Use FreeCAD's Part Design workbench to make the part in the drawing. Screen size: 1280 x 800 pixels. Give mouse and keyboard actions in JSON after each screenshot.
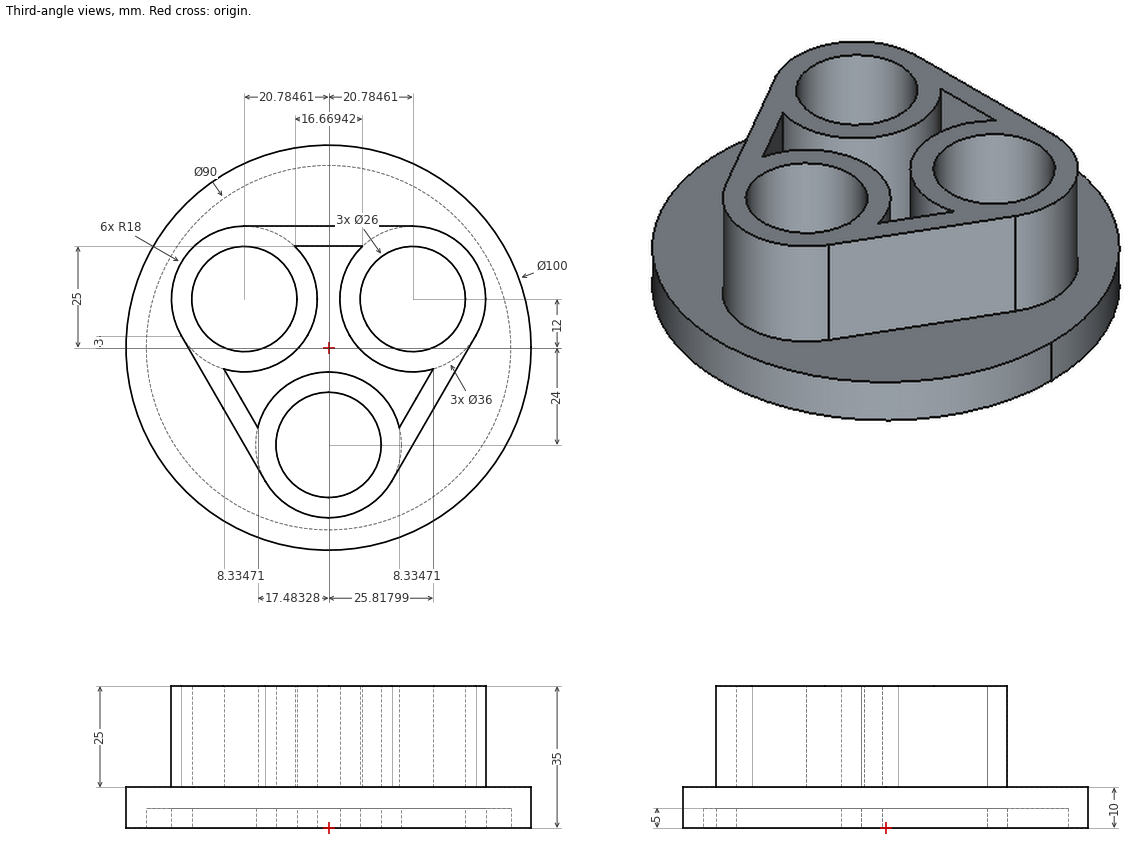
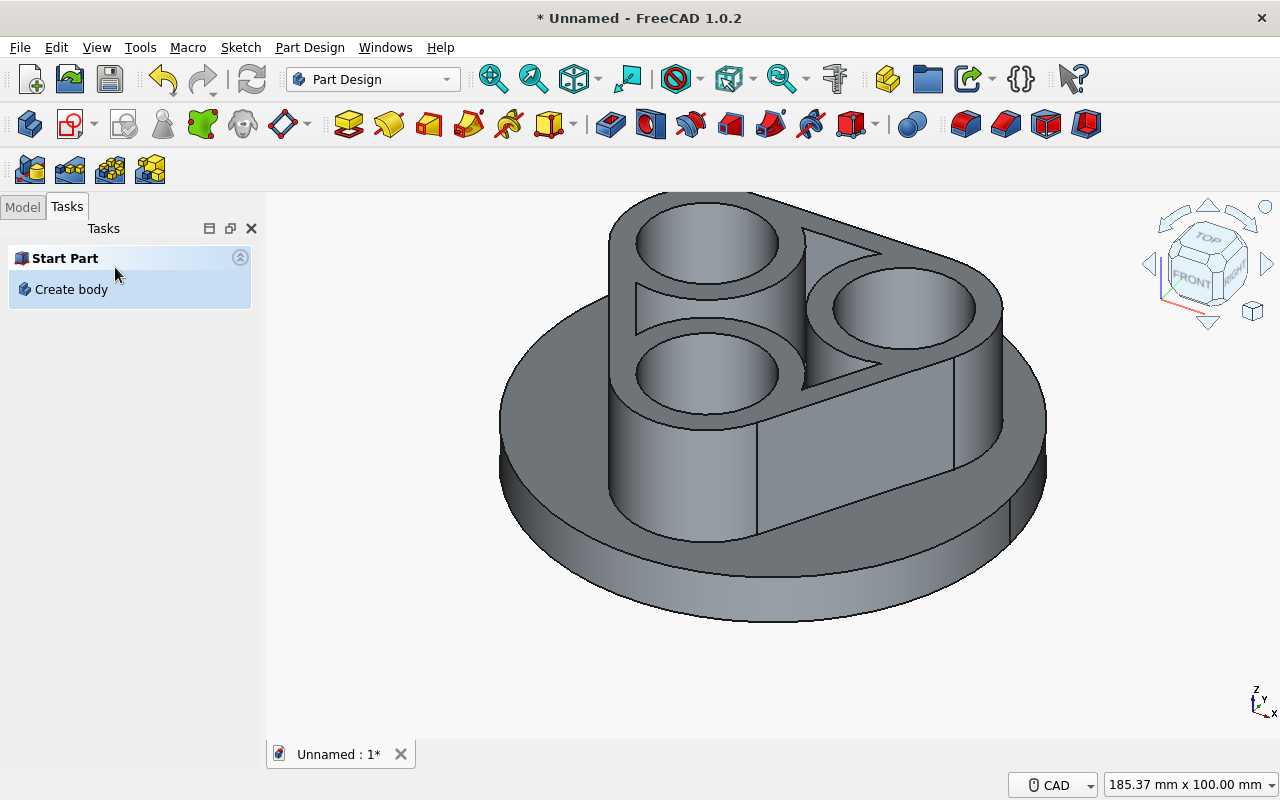
{"action": "left_click", "coordinate": [494, 80]}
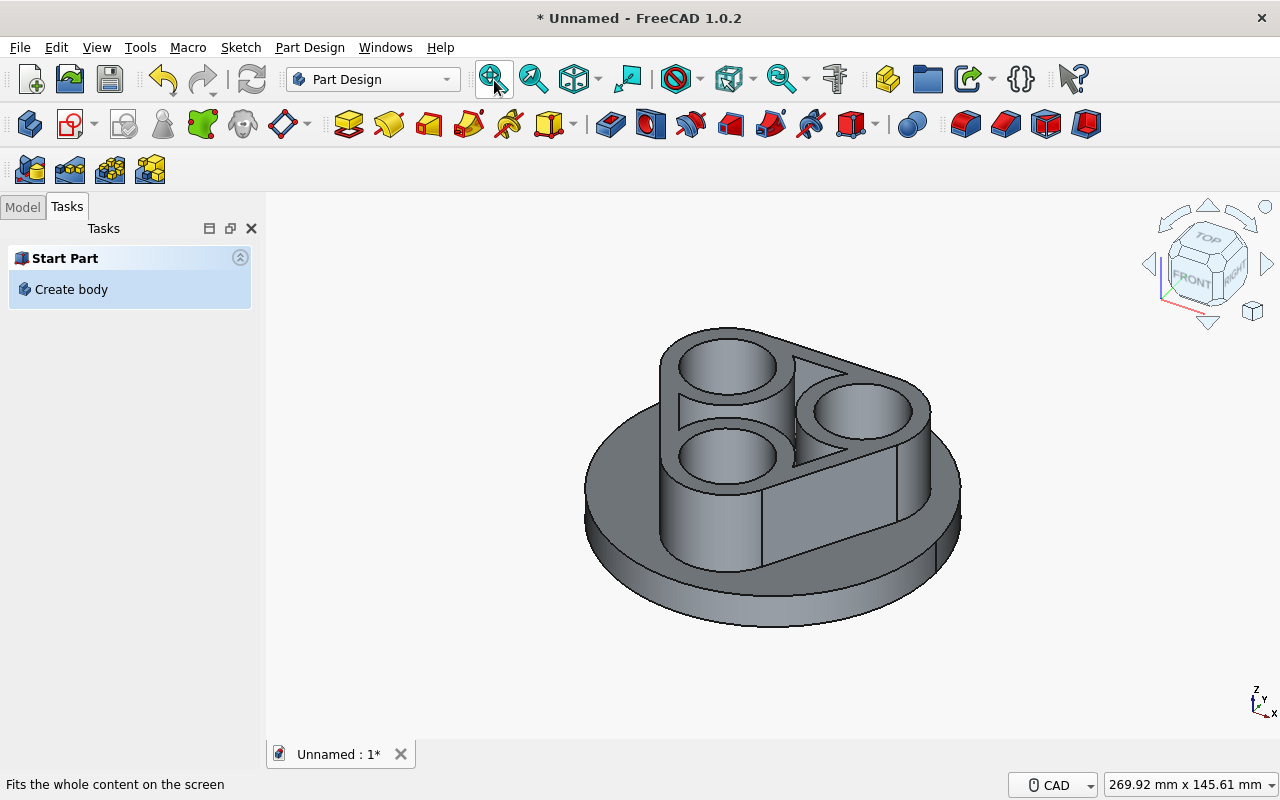
{"action": "key", "text": "5"}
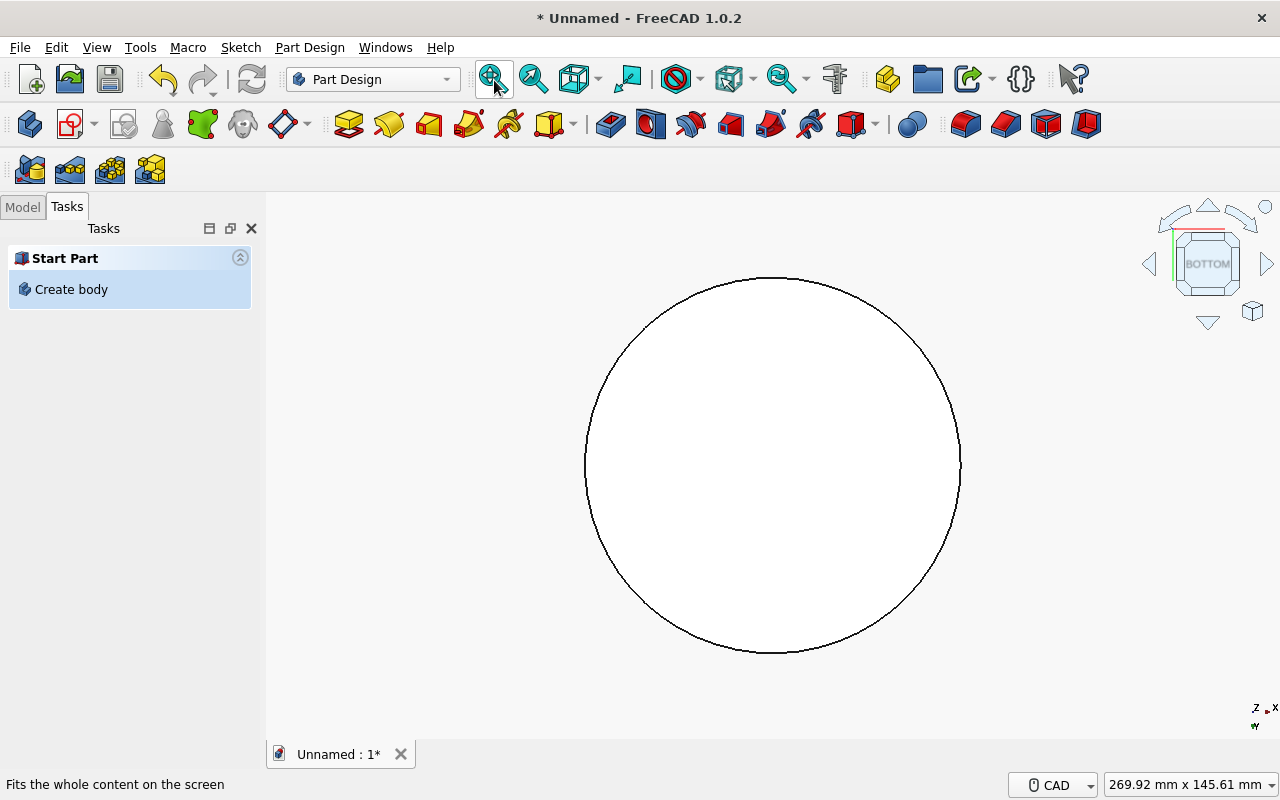
{"action": "left_click", "coordinate": [773, 464]}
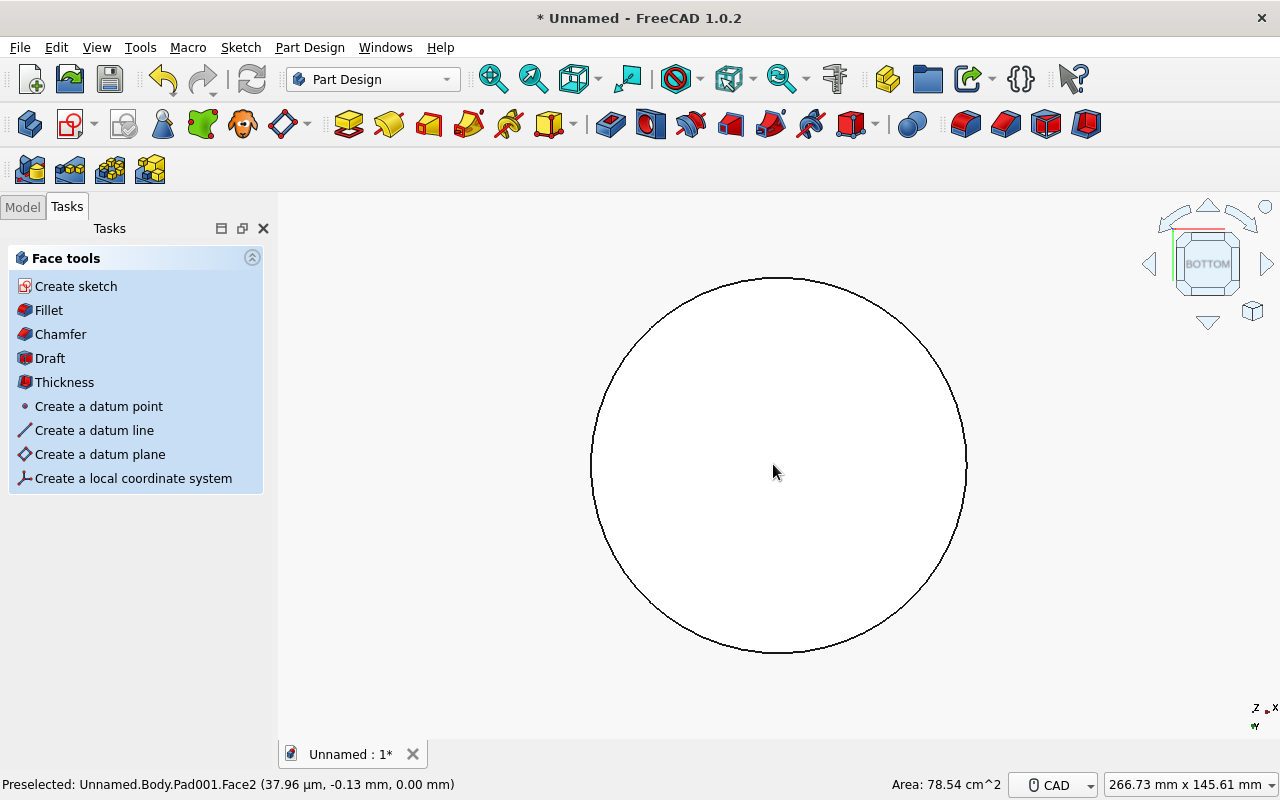
{"action": "left_click", "coordinate": [70, 124]}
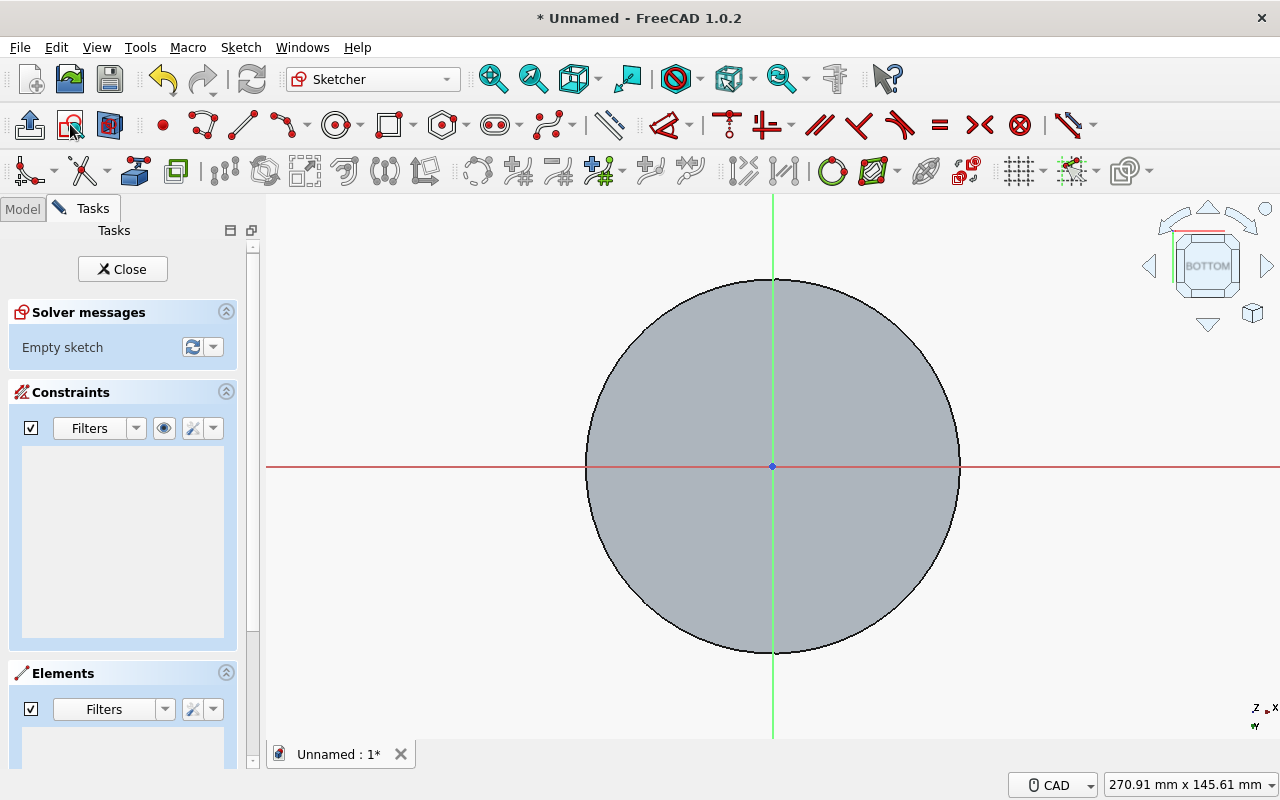
{"action": "left_click", "coordinate": [336, 126]}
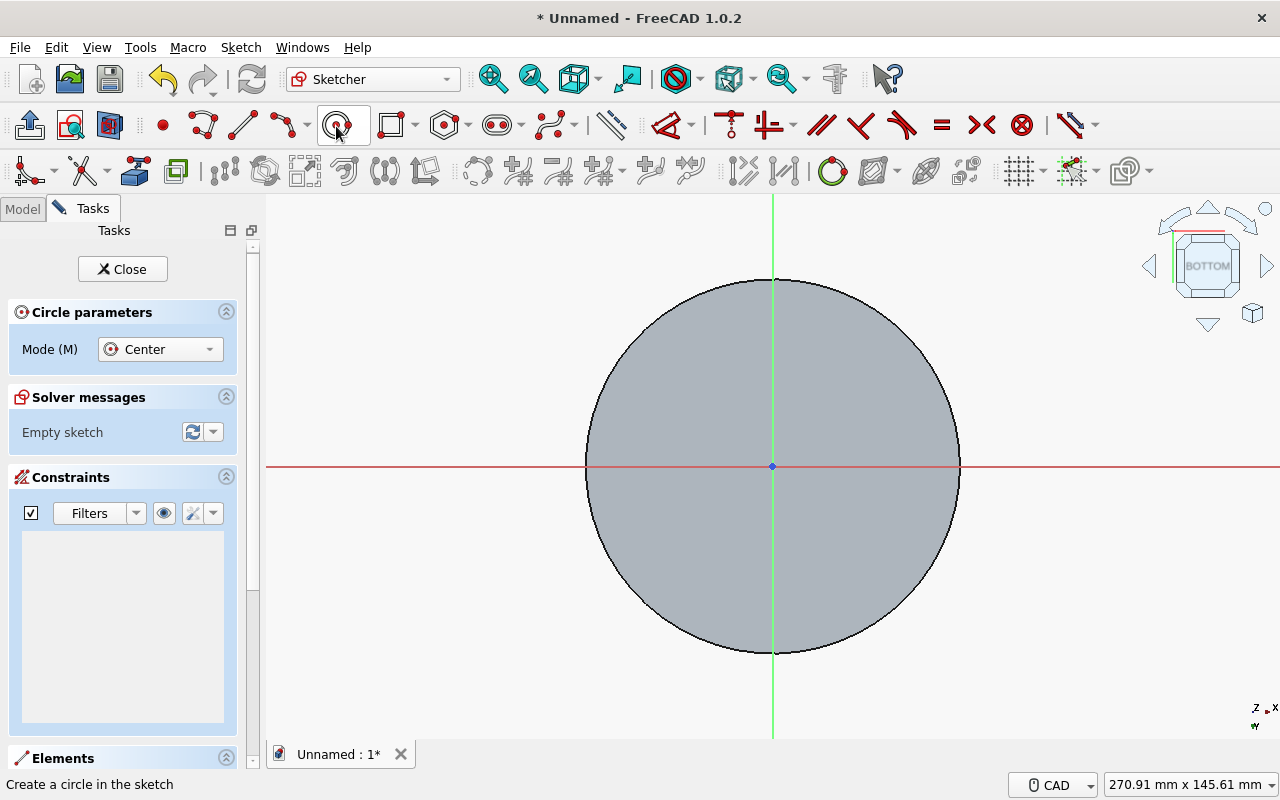
{"action": "left_click", "coordinate": [773, 466]}
{"action": "left_click", "coordinate": [892, 347]}
{"action": "key", "text": "Escape"}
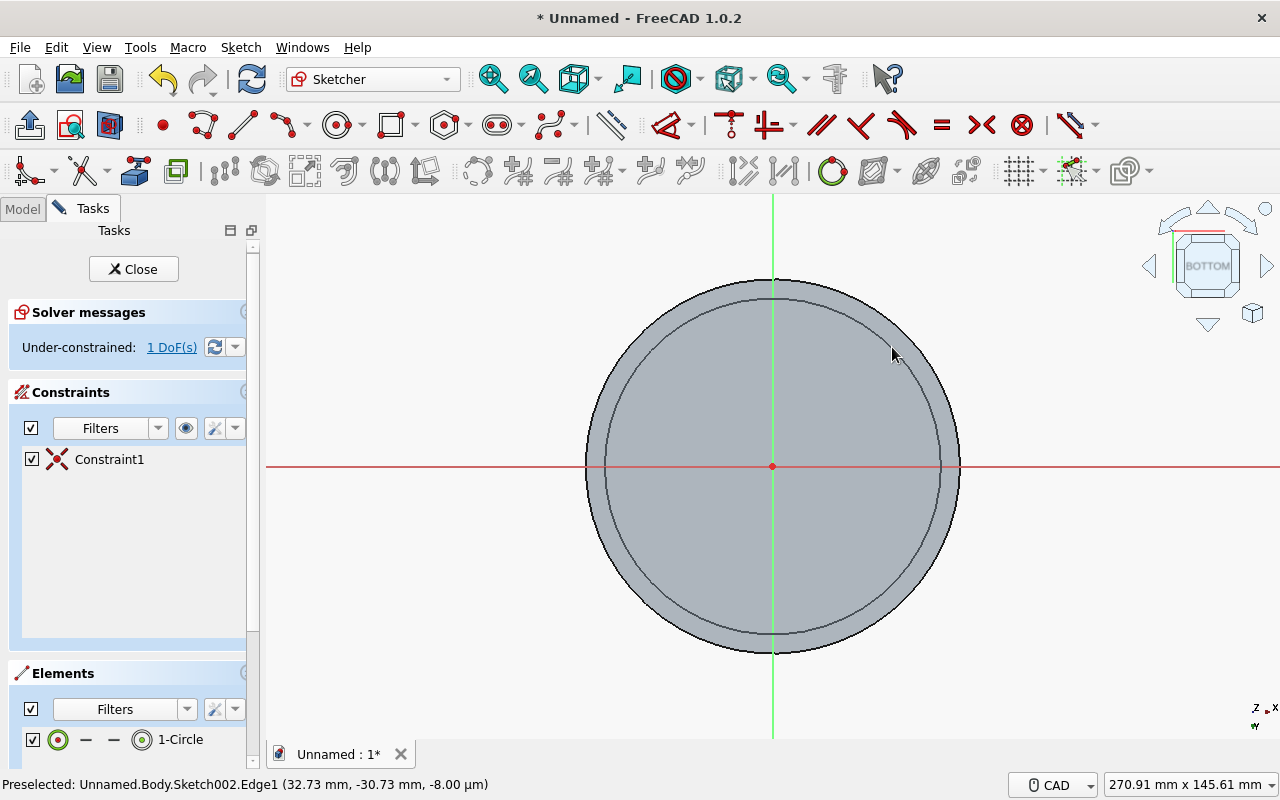
{"action": "left_click", "coordinate": [666, 126]}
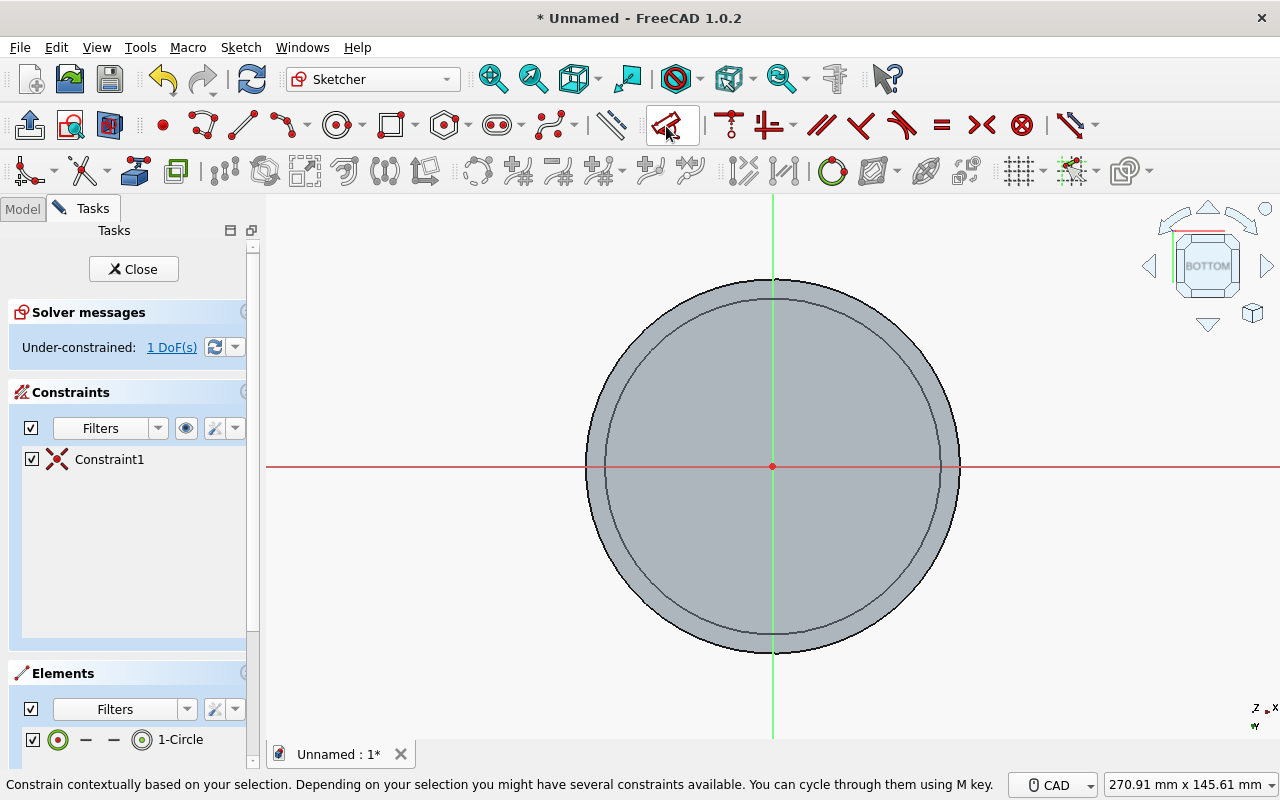
{"action": "left_click", "coordinate": [891, 347]}
{"action": "left_click", "coordinate": [913, 324]}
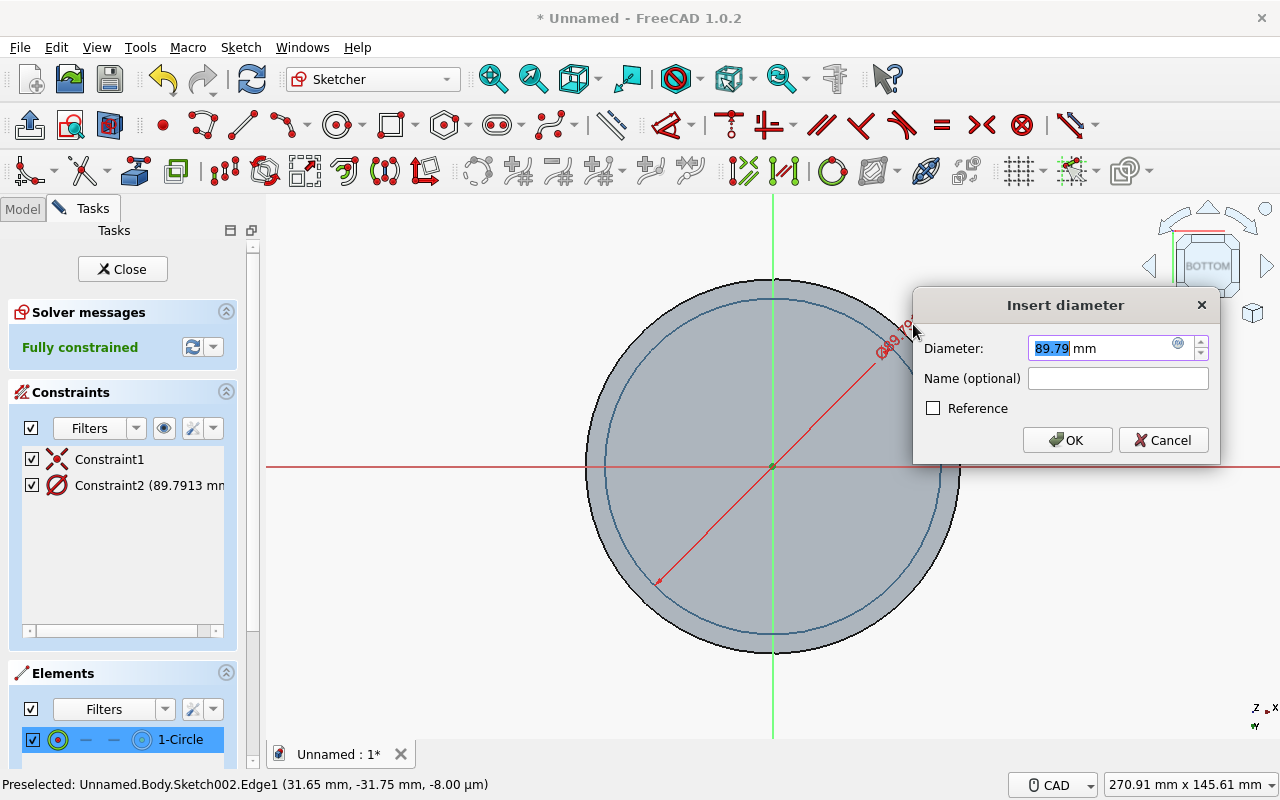
{"action": "type", "text": "90"}
{"action": "key", "text": "Return"}
{"action": "key", "text": "Escape"}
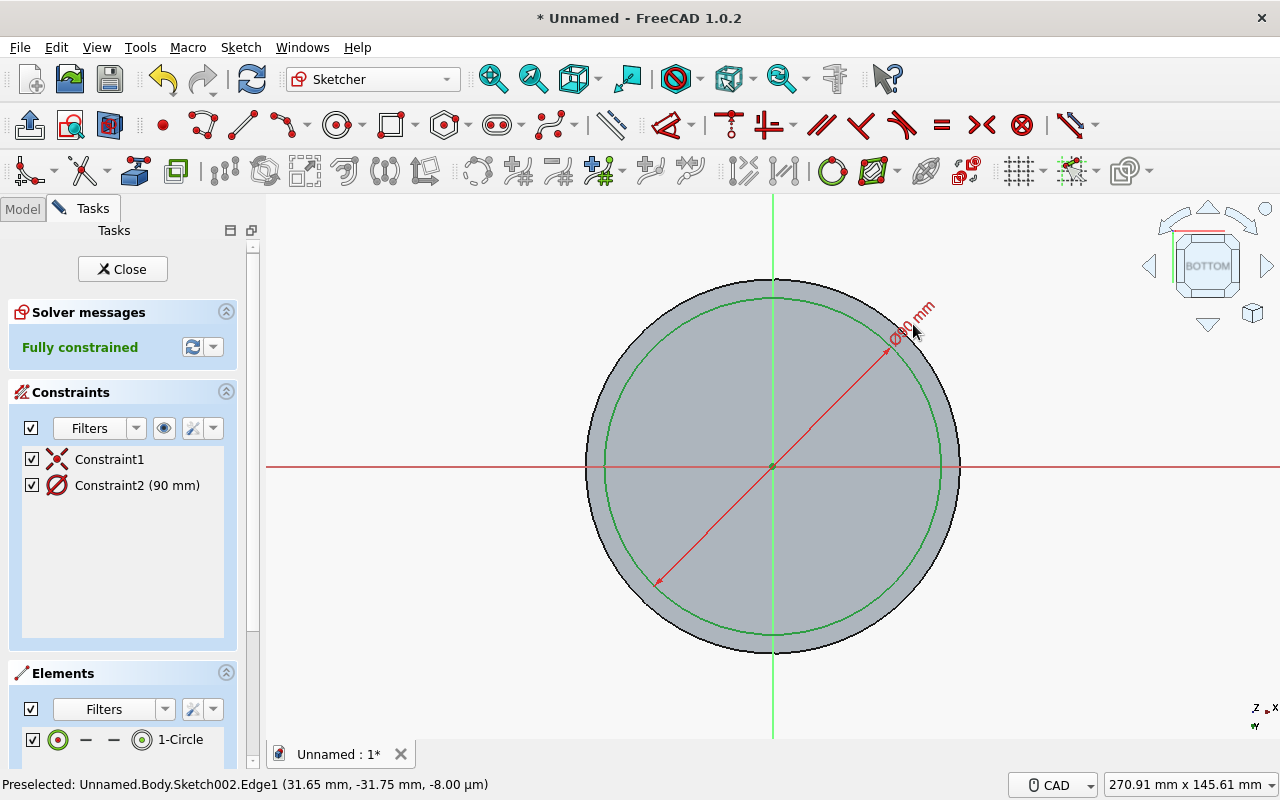
{"action": "left_click", "coordinate": [123, 269]}